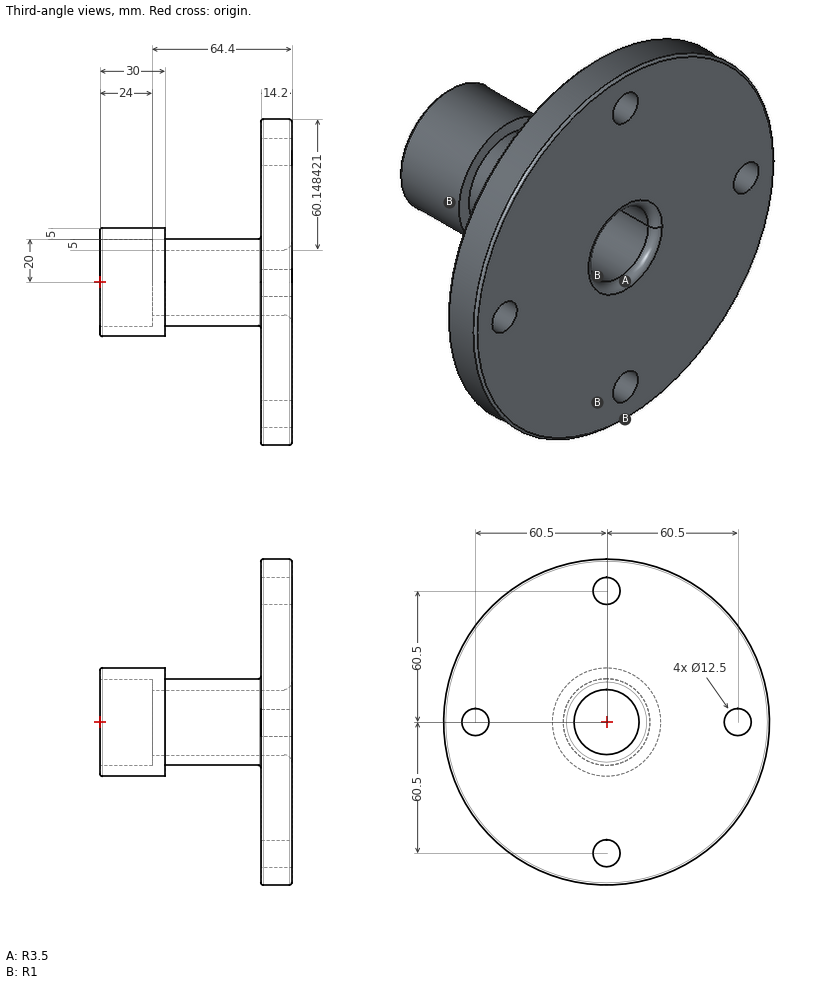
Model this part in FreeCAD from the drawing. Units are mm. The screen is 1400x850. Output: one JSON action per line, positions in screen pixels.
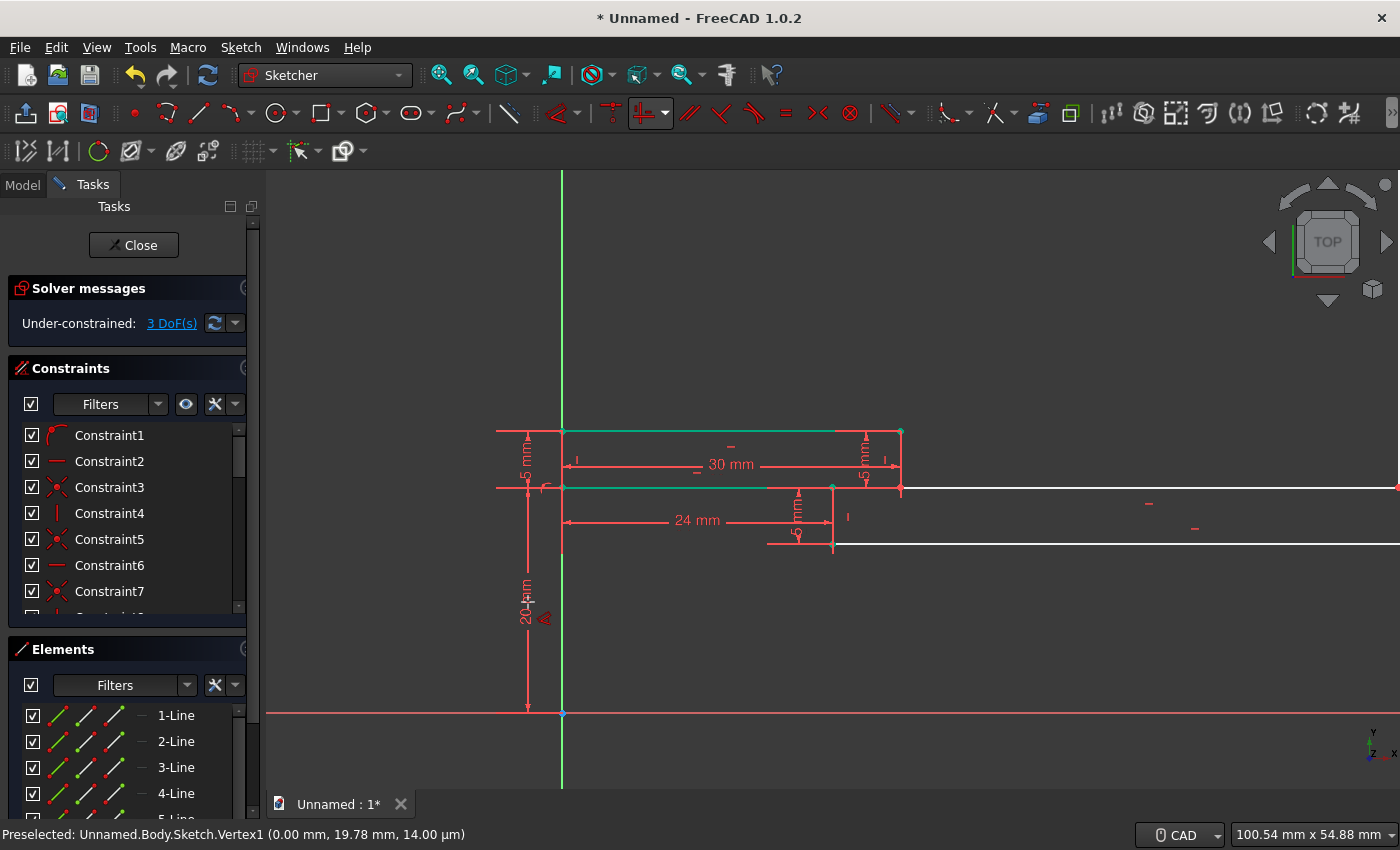
{"action": "left_click", "coordinate": [1051, 544]}
{"action": "left_click", "coordinate": [1034, 578]}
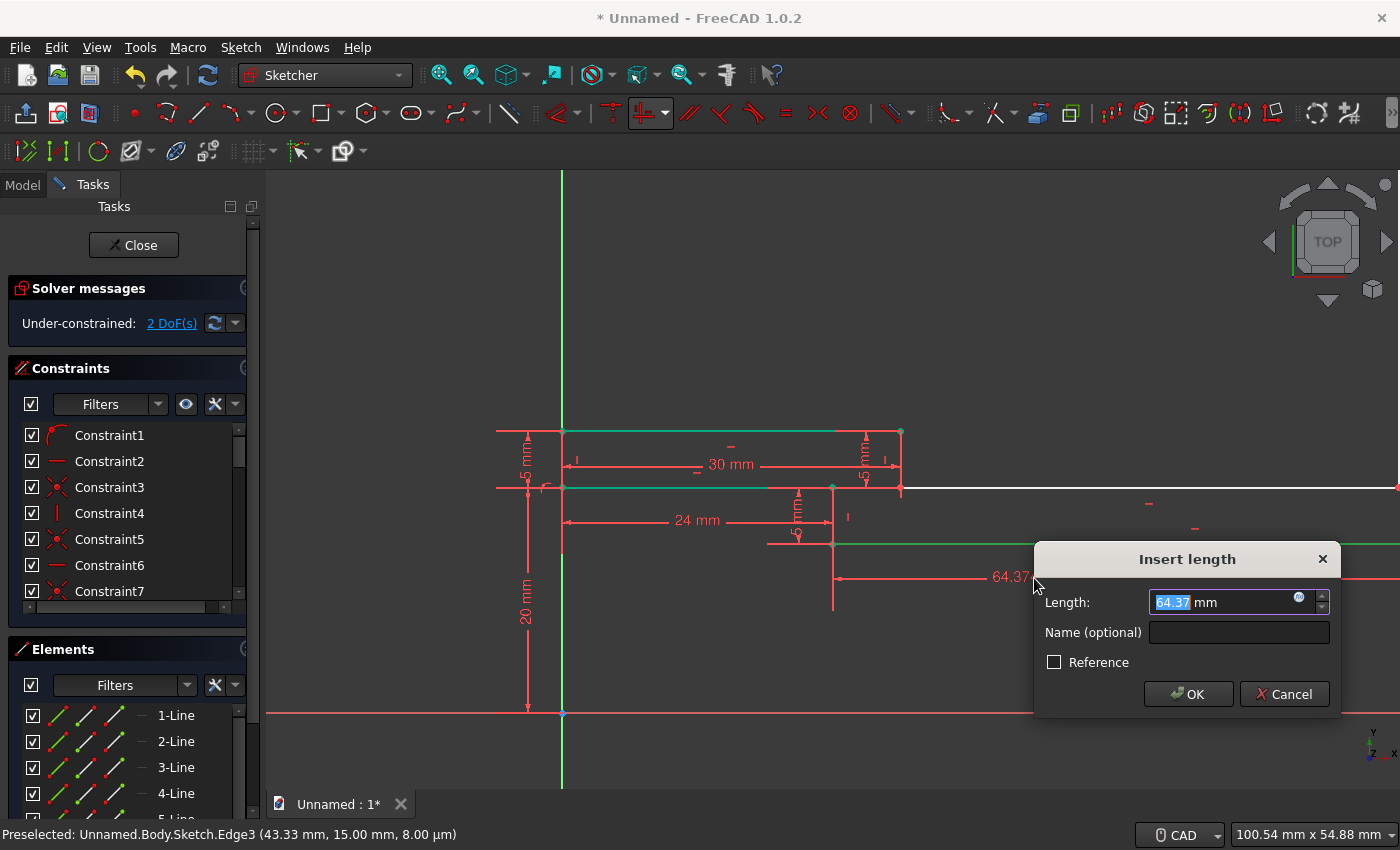
{"action": "type", "text": "64.4"}
{"action": "key", "text": "Return"}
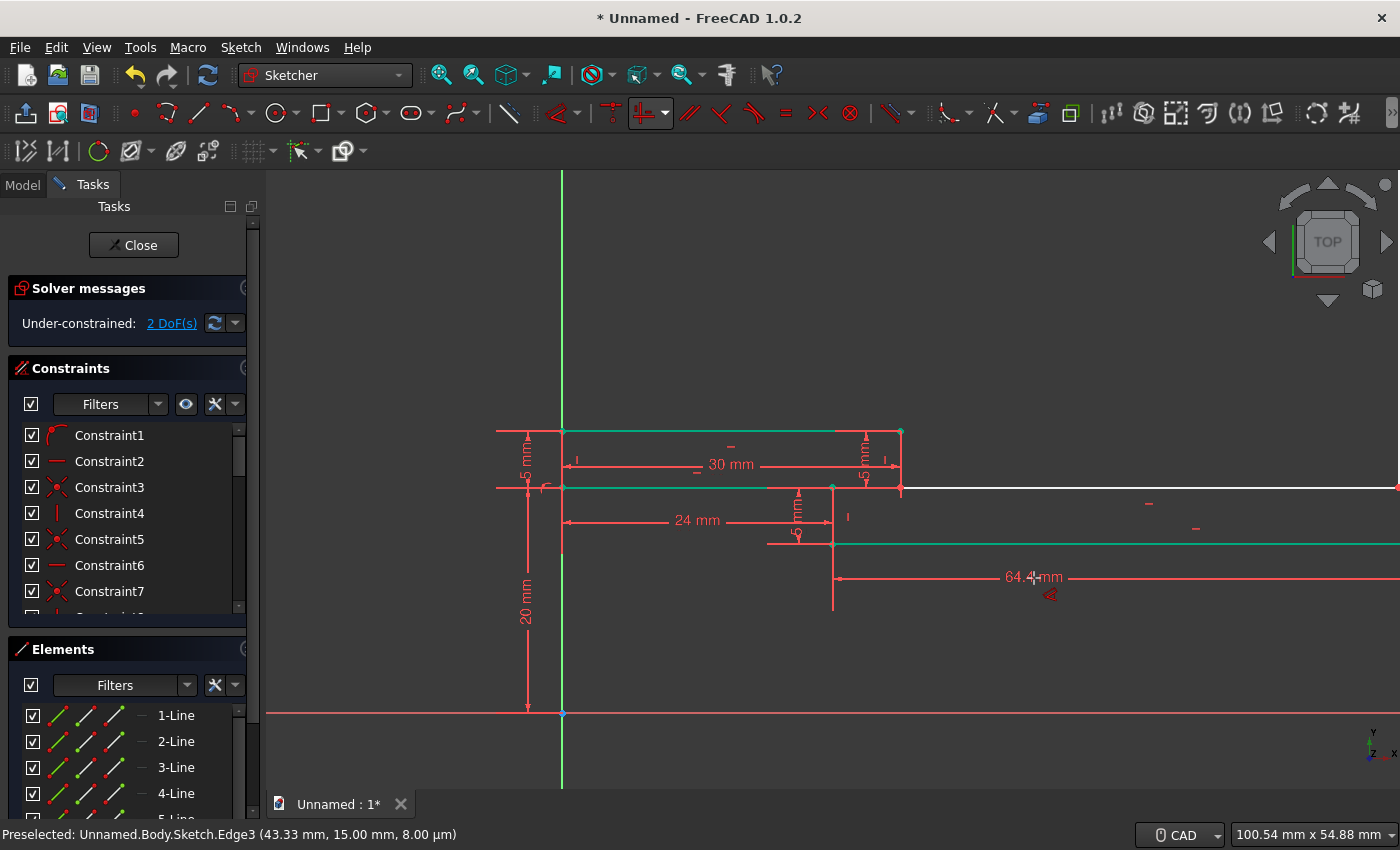
{"action": "scroll", "coordinate": [523, 634], "scroll_direction": "down", "scroll_amount": 4}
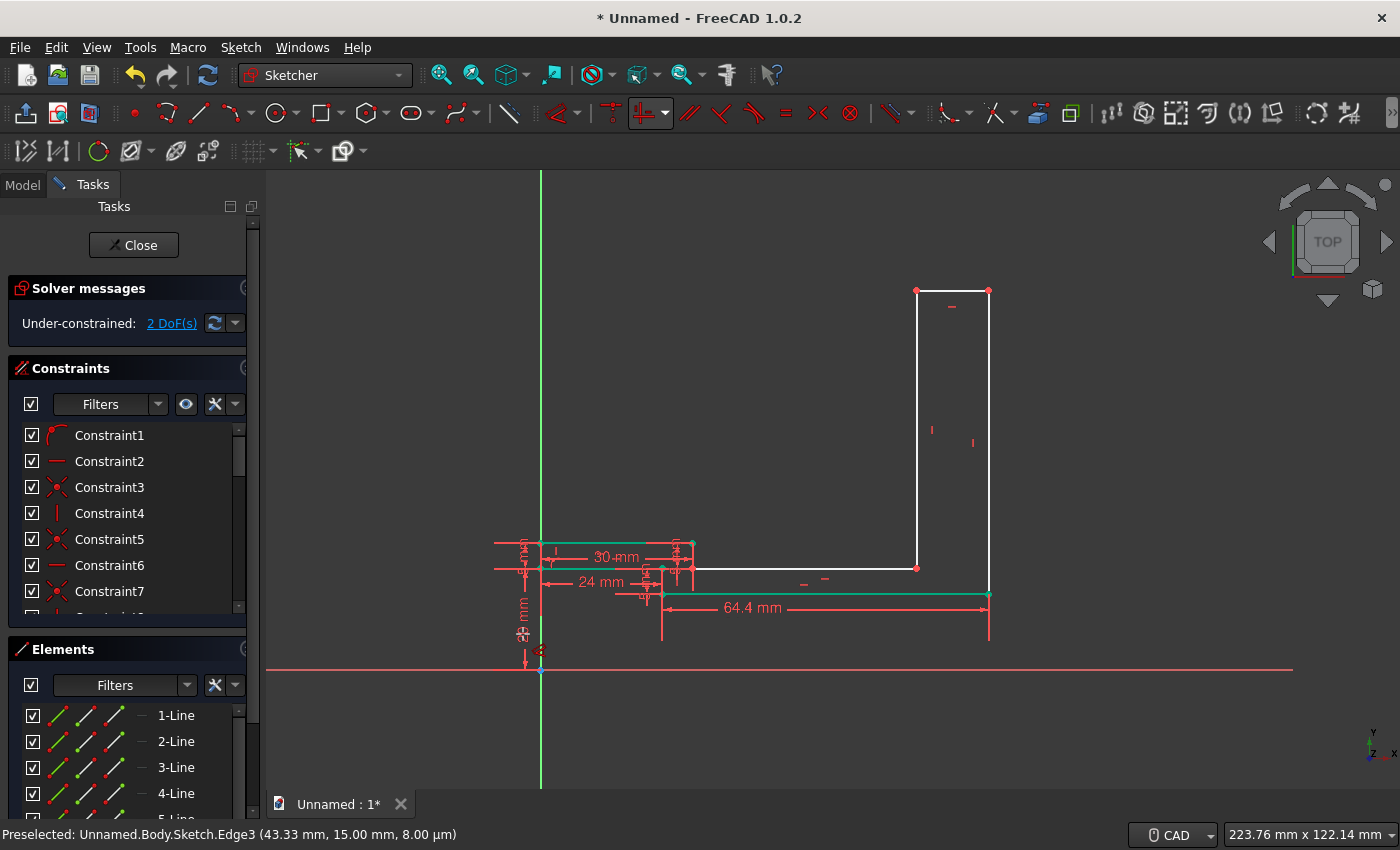
{"action": "left_click", "coordinate": [967, 291]}
{"action": "left_click", "coordinate": [953, 257]}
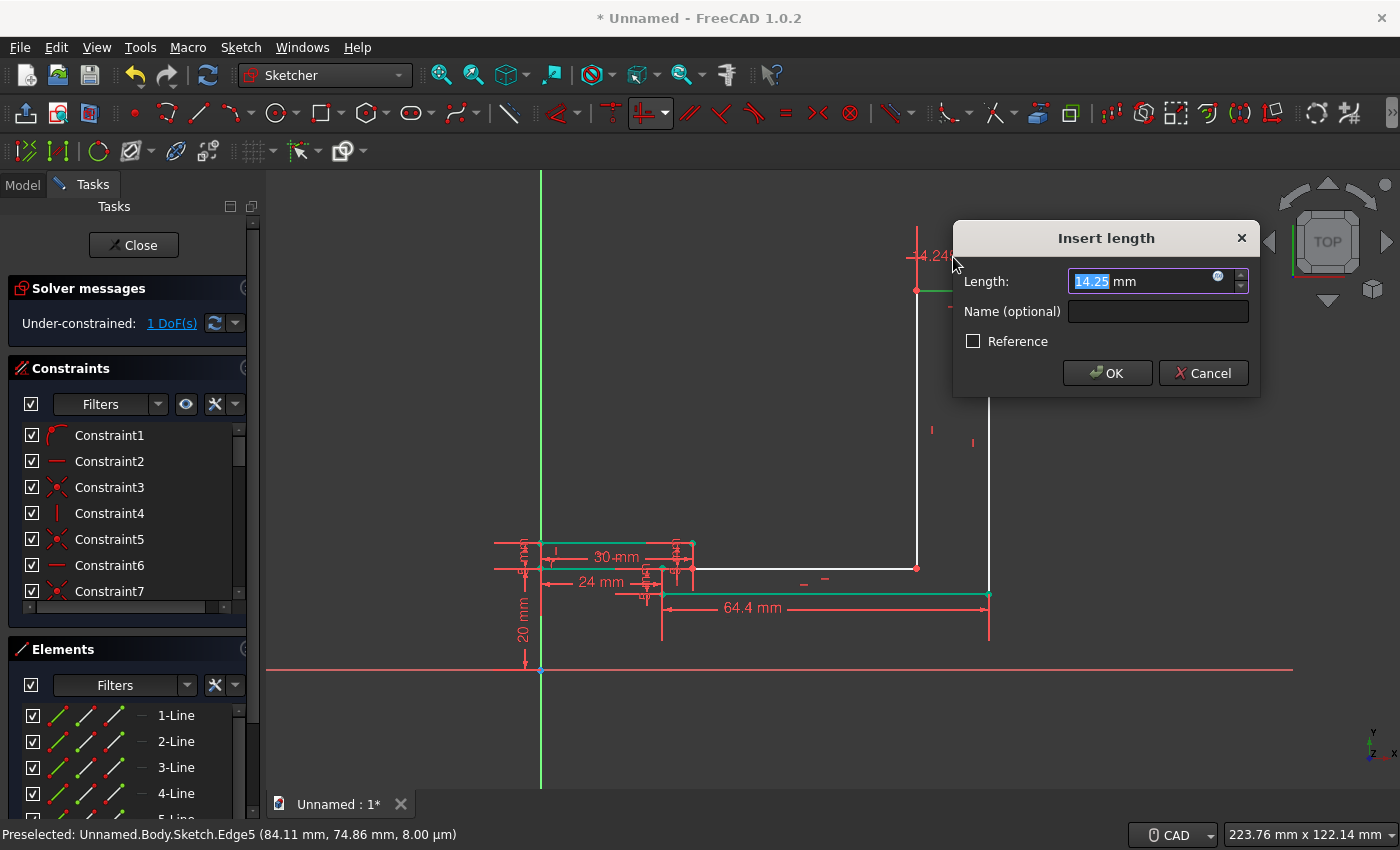
{"action": "type", "text": "14.2"}
{"action": "key", "text": "Return"}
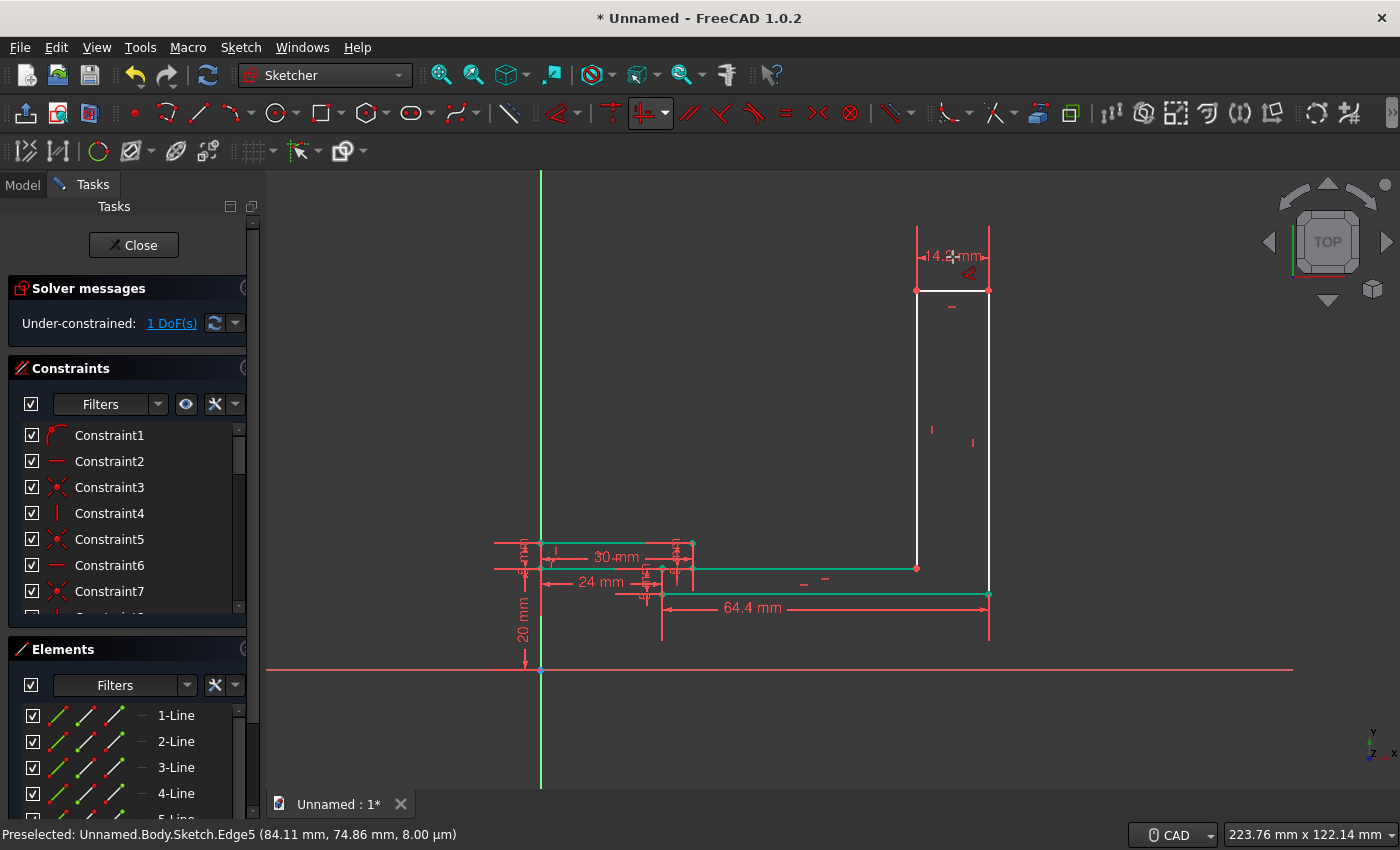
{"action": "left_click", "coordinate": [989, 503]}
{"action": "left_click", "coordinate": [1023, 442]}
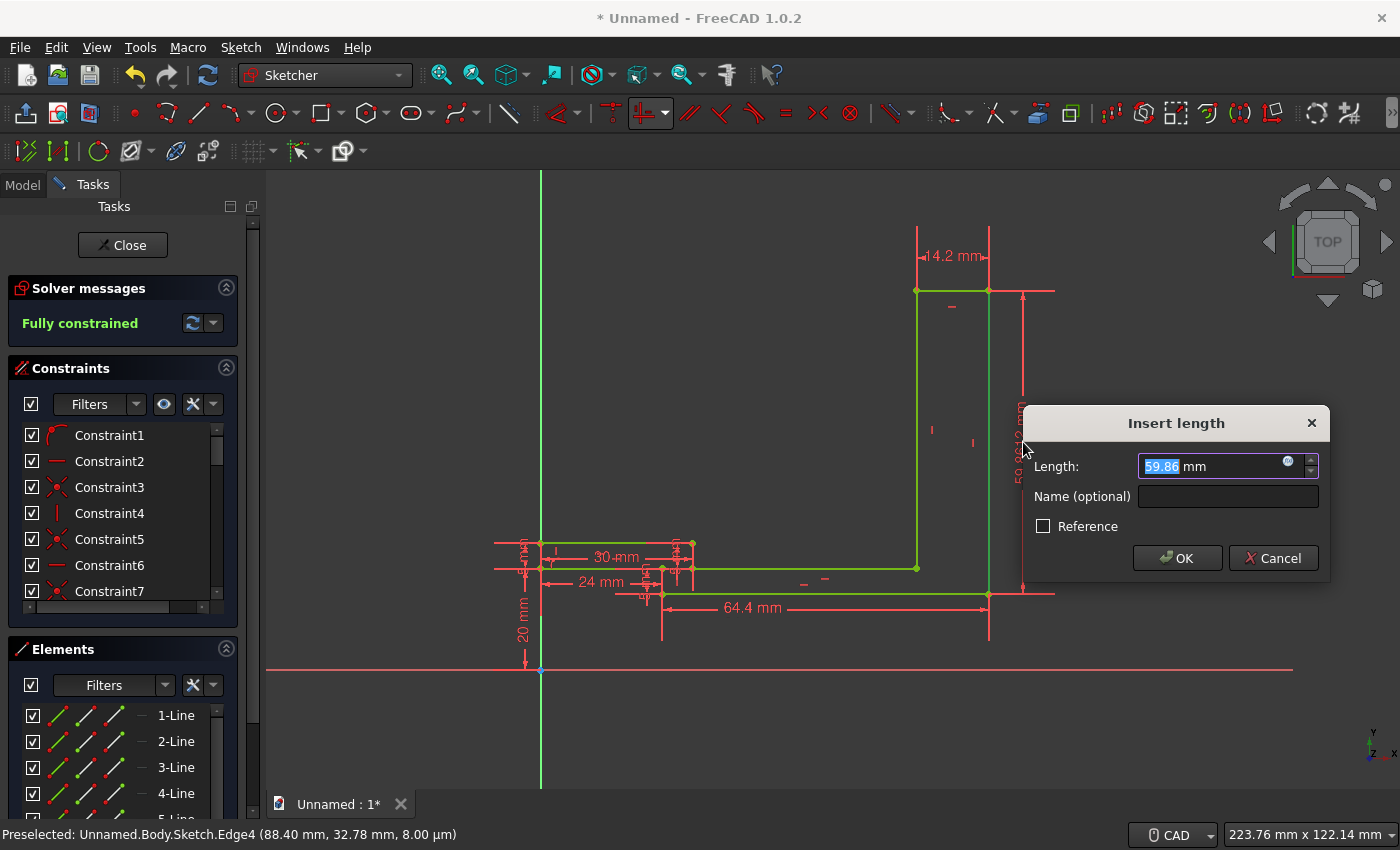
{"action": "type", "text": "60.148421"}
{"action": "key", "text": "Return"}
{"action": "key", "text": "Escape"}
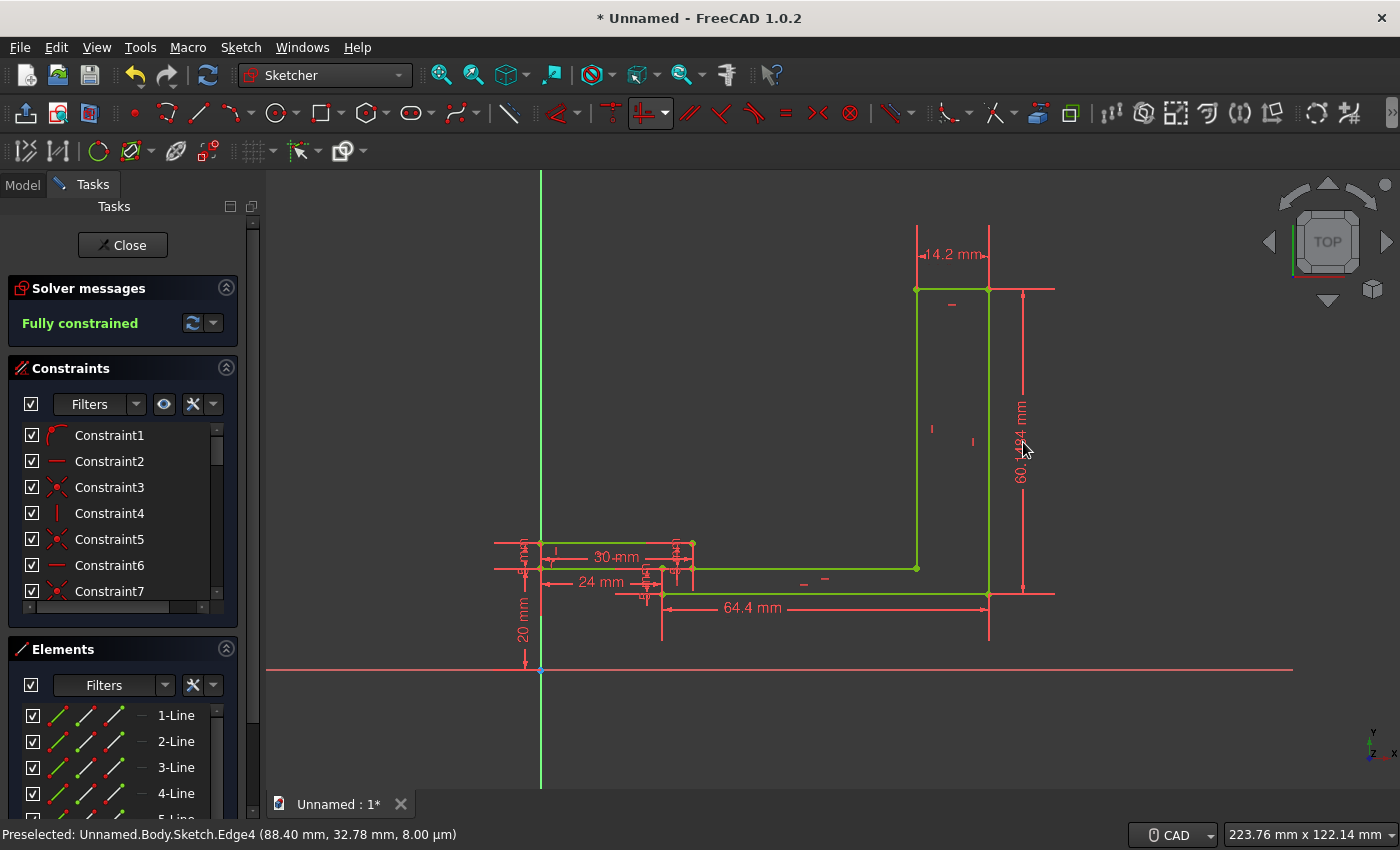
{"action": "left_click", "coordinate": [123, 245]}